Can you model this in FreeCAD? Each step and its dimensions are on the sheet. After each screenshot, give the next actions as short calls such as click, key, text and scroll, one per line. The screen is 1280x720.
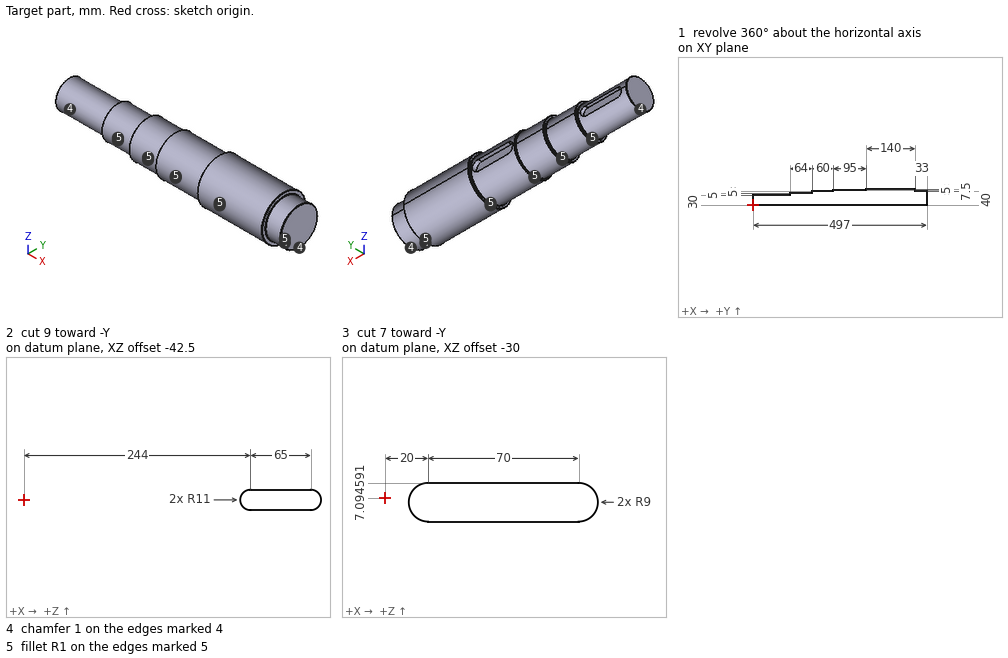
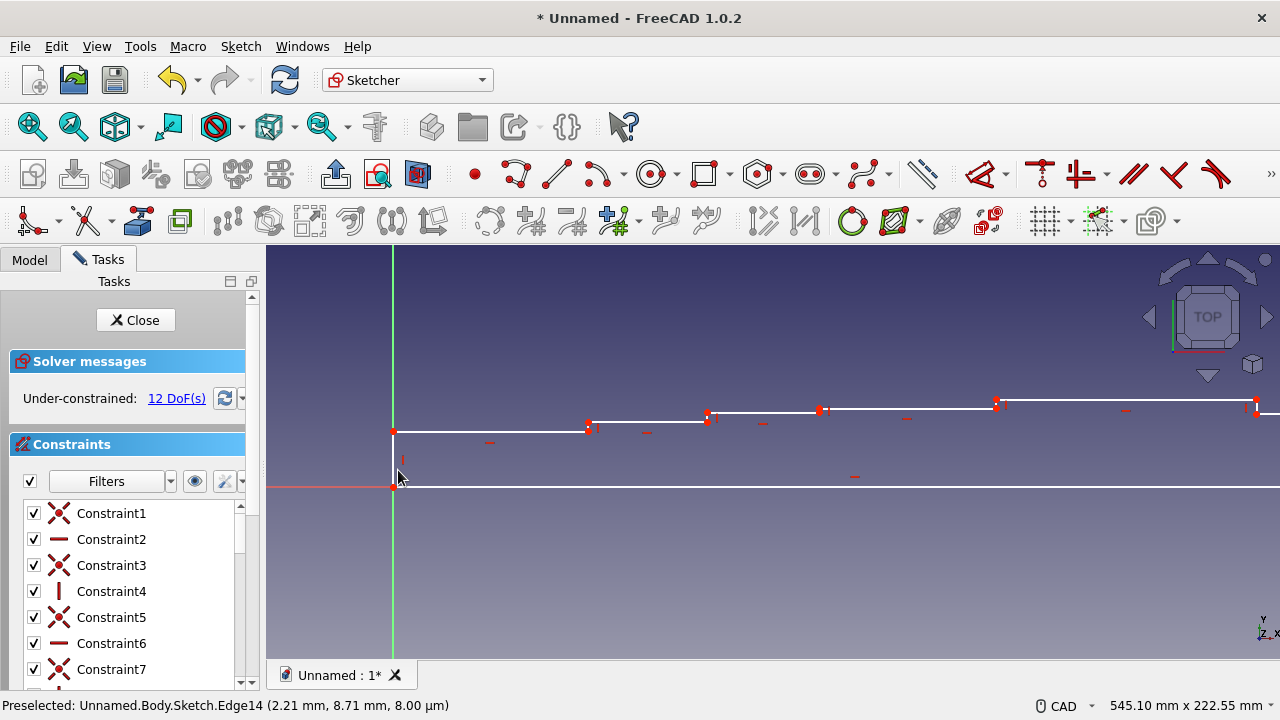
scroll(996, 404, up, 8)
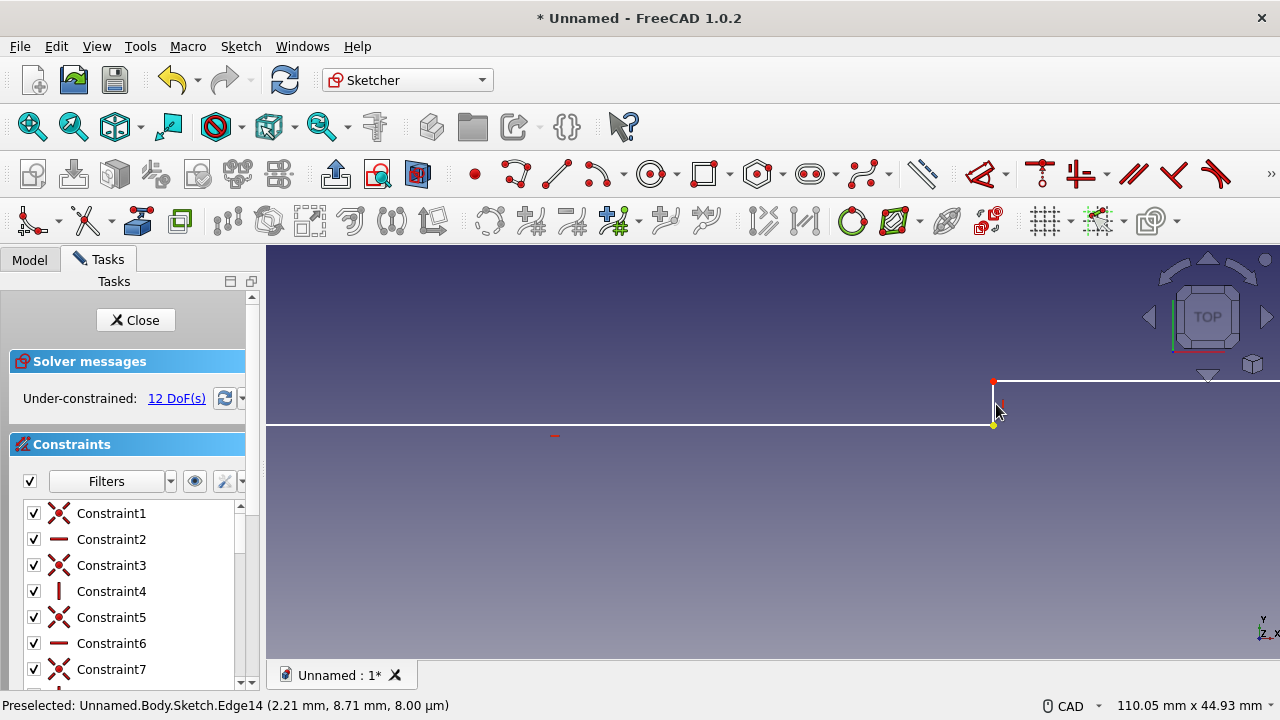
click(993, 403)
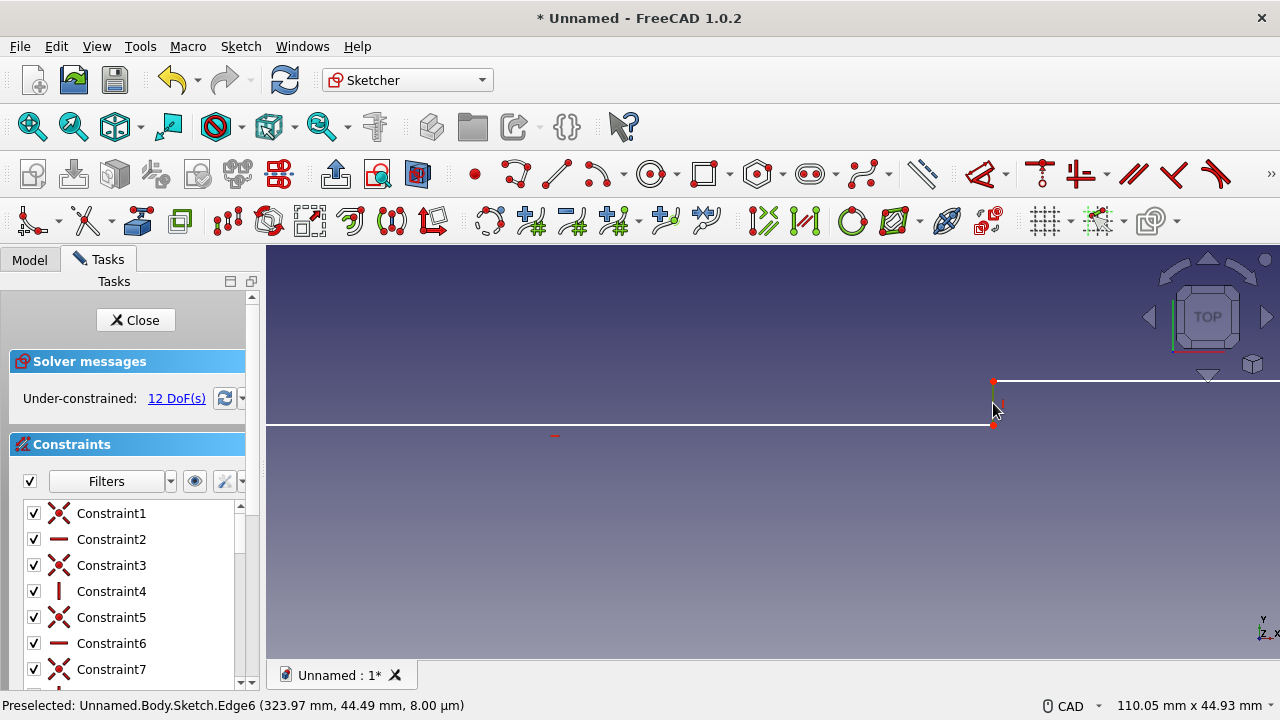
click(1006, 174)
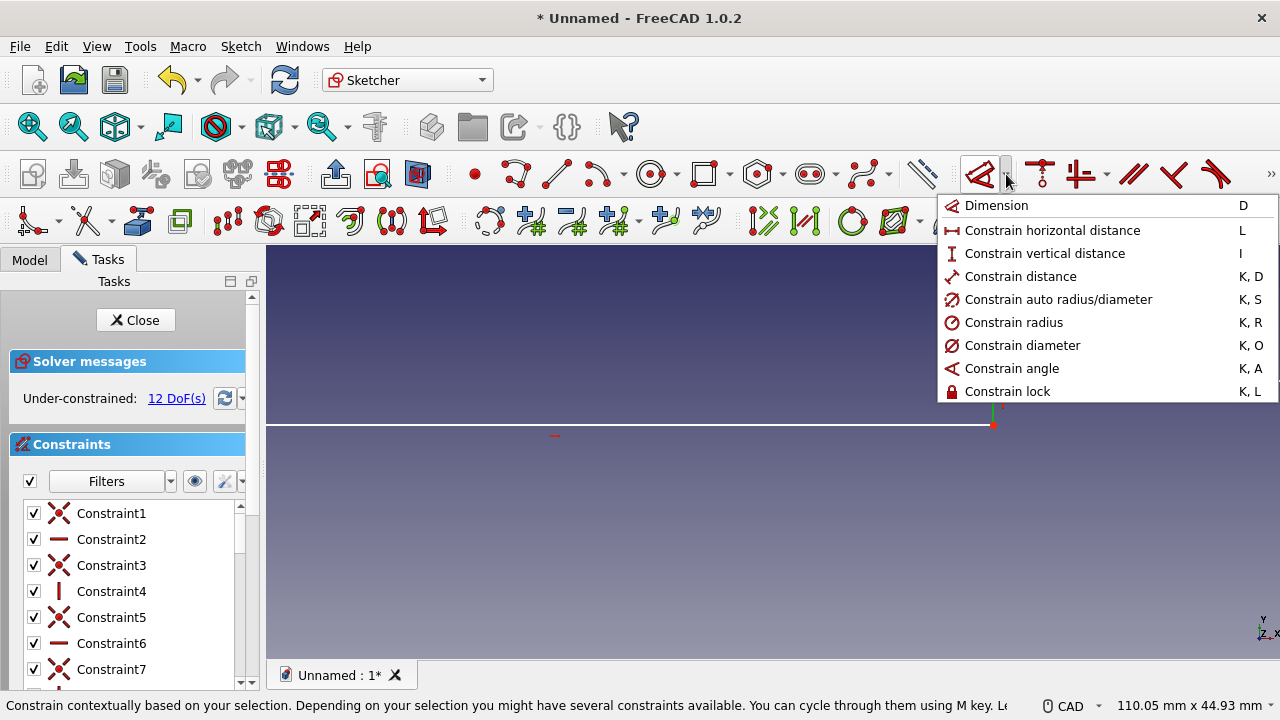
click(1108, 254)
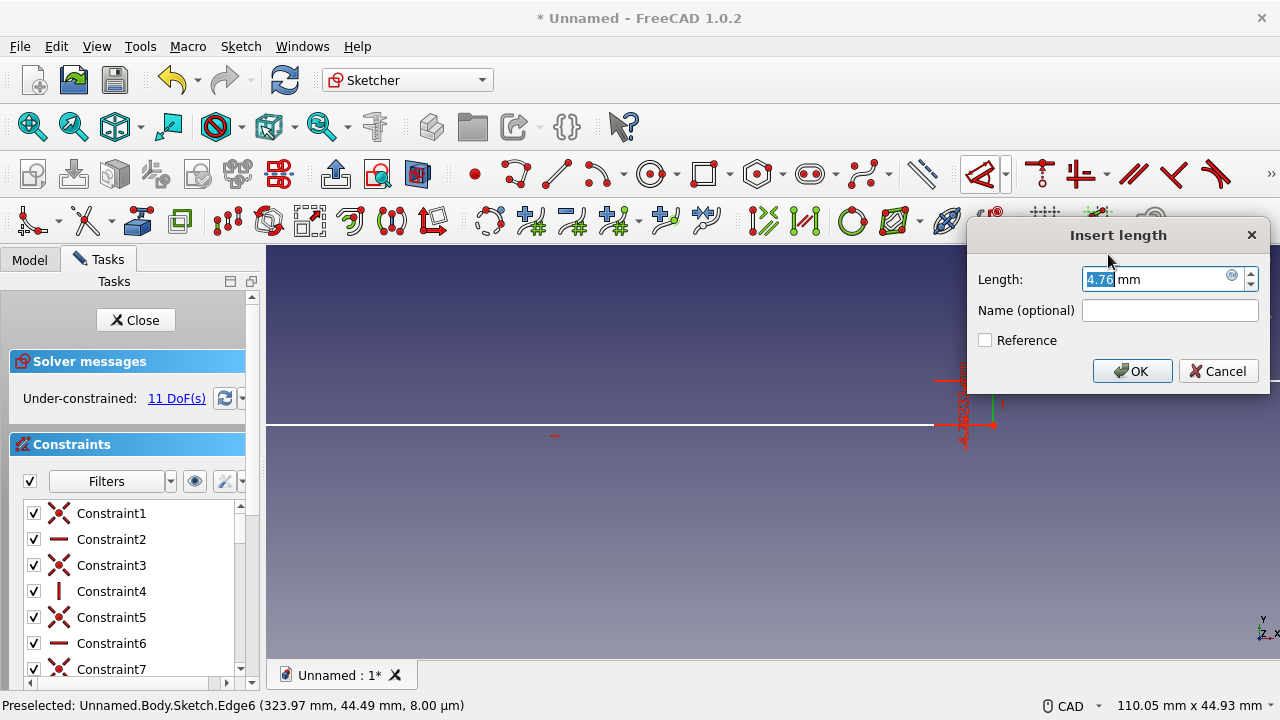
text(5)
key(Return)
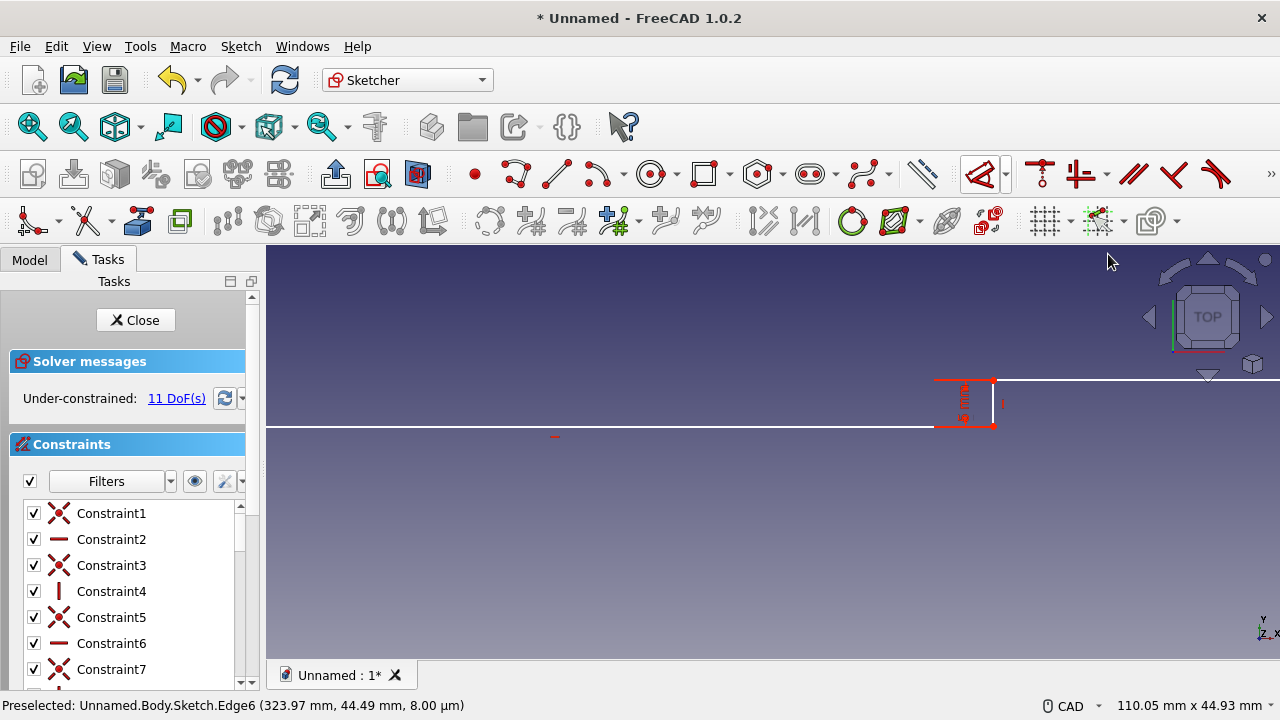
scroll(768, 430, down, 10)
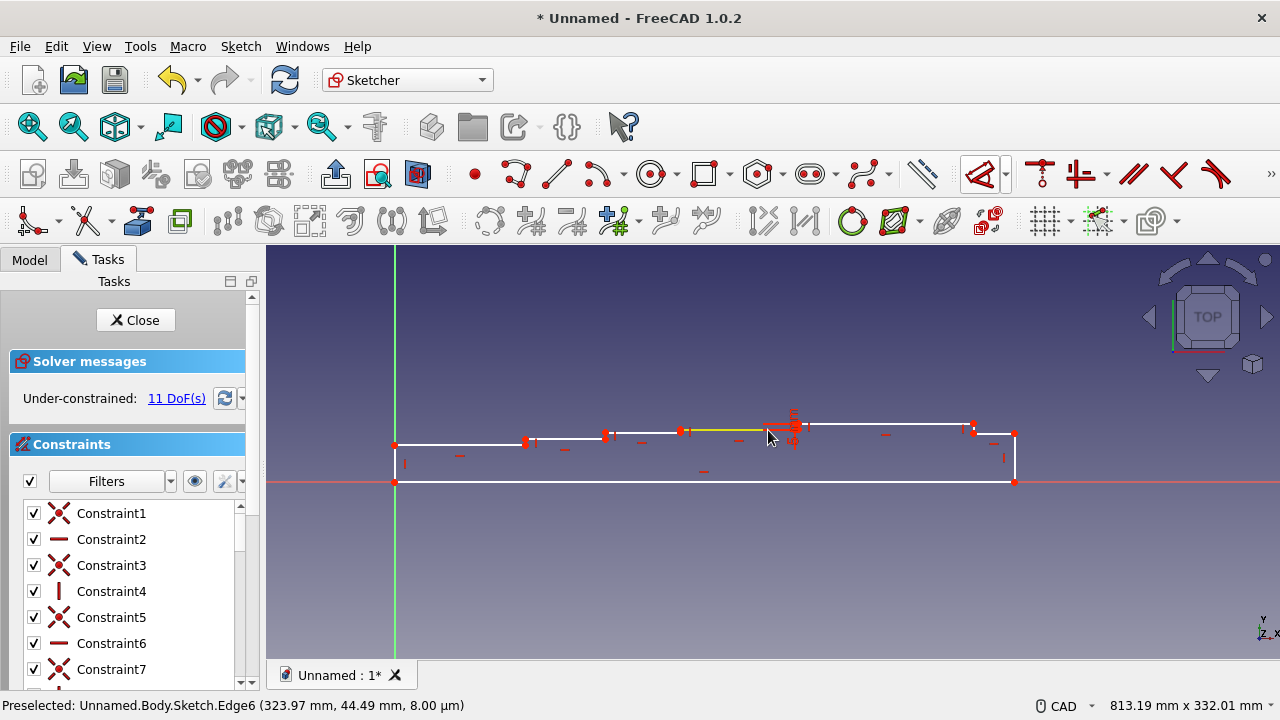
scroll(605, 435, up, 10)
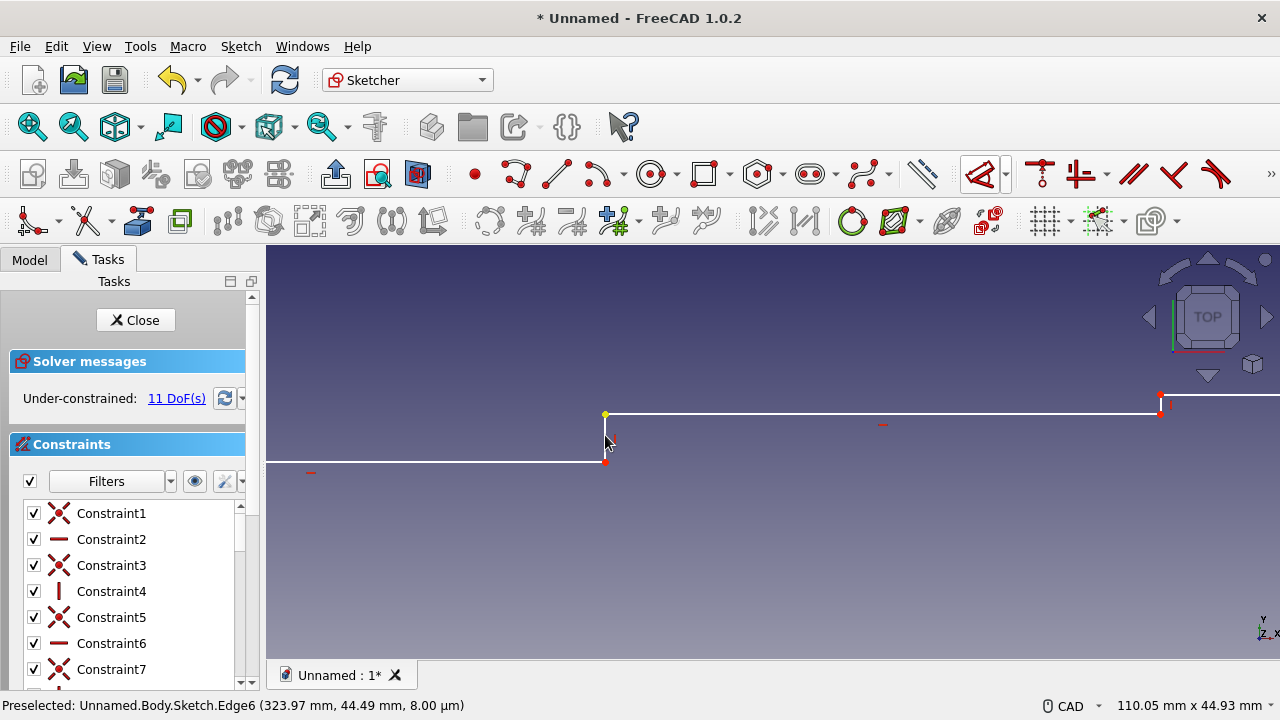
click(605, 429)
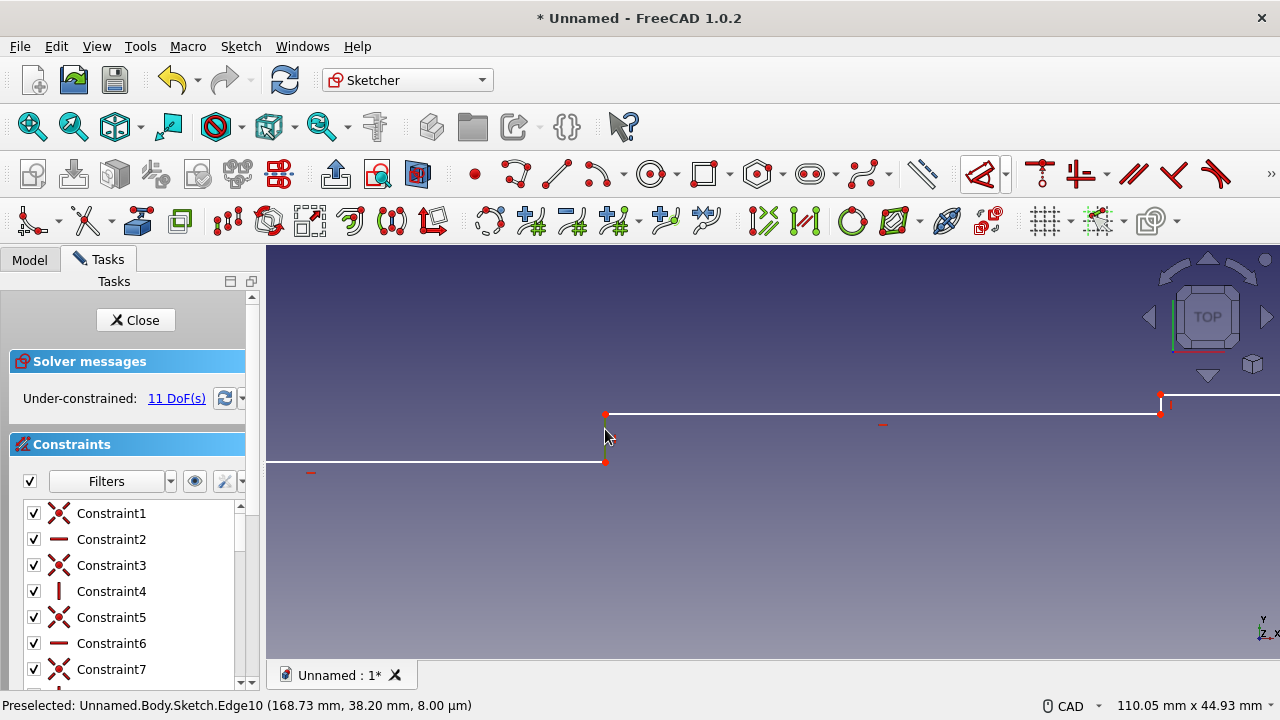
click(1006, 174)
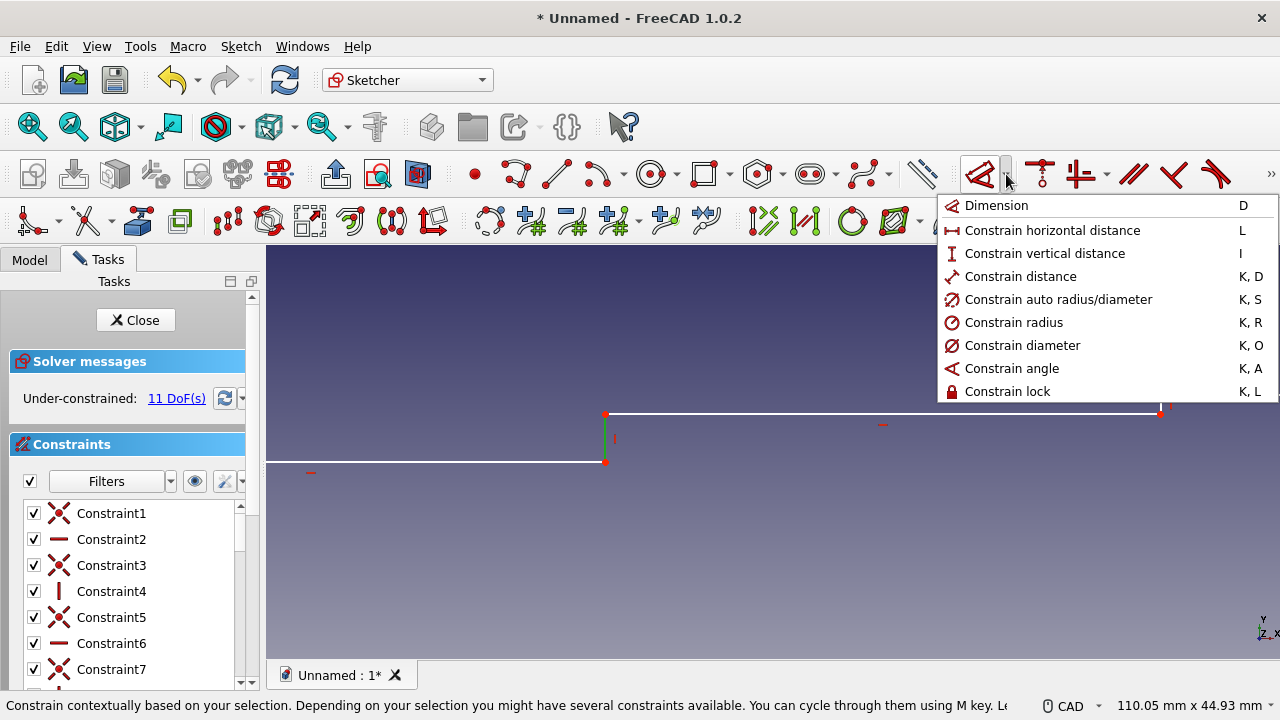
click(1108, 254)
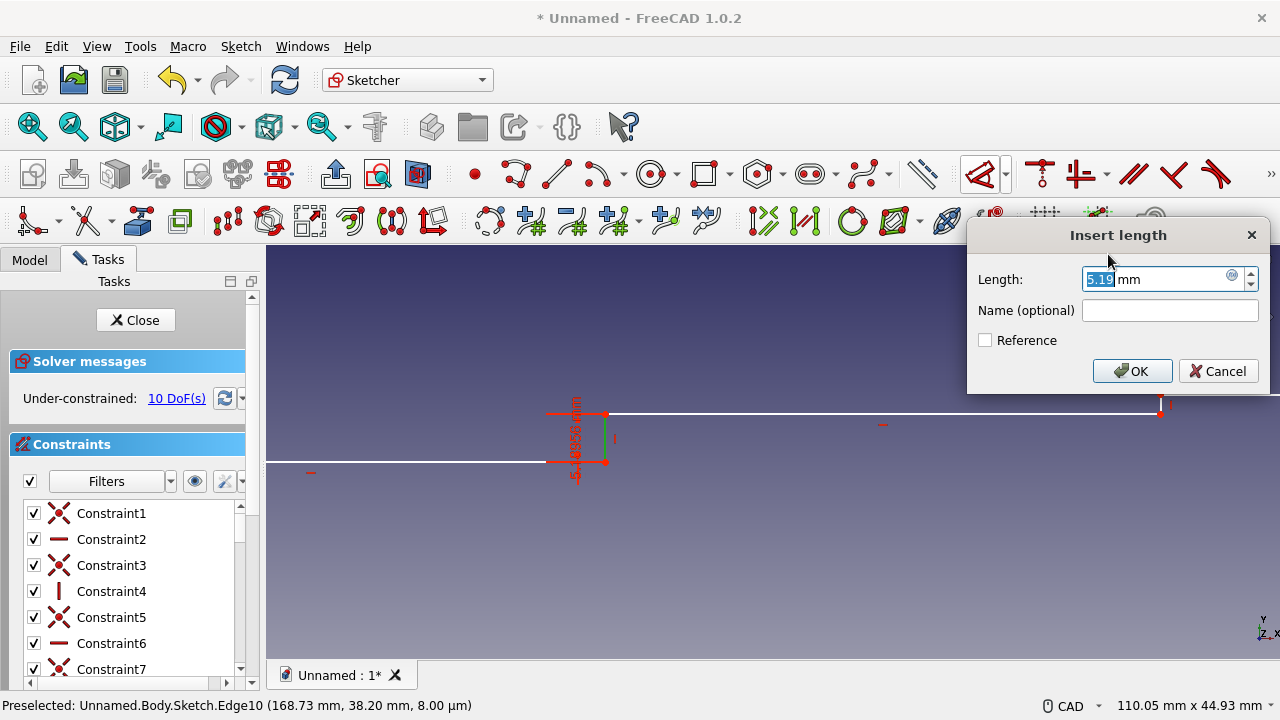
text(5)
key(Return)